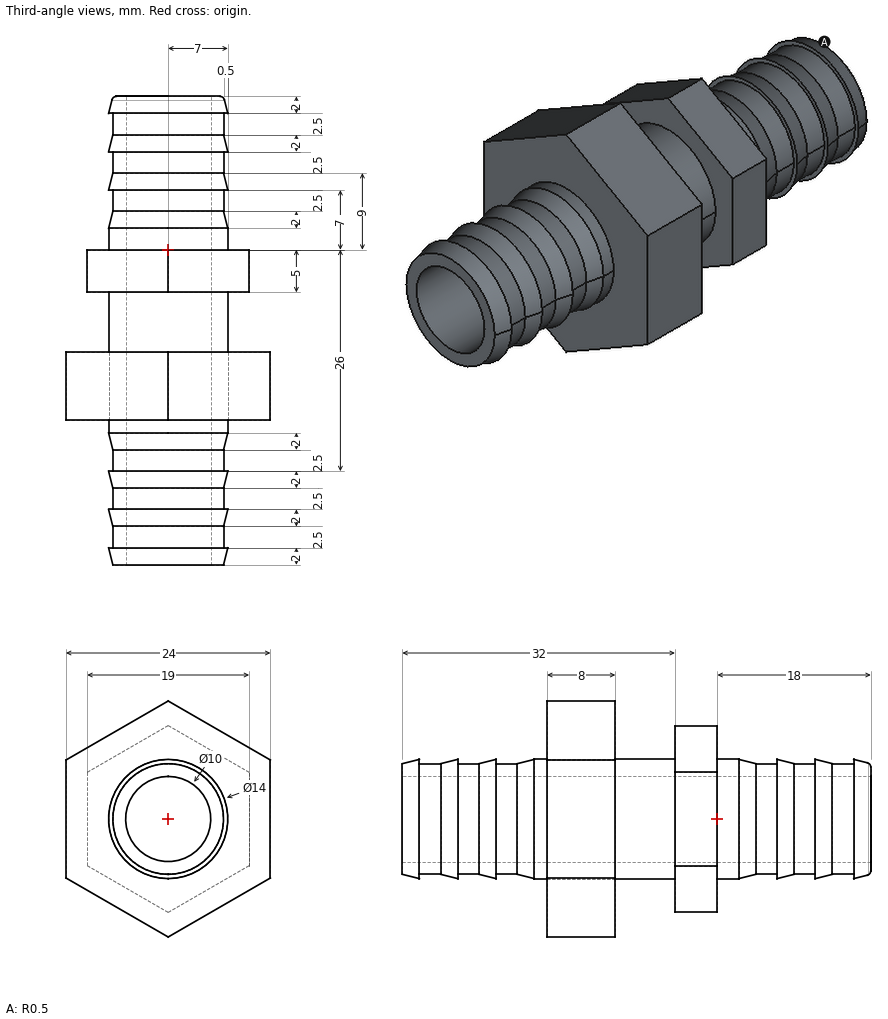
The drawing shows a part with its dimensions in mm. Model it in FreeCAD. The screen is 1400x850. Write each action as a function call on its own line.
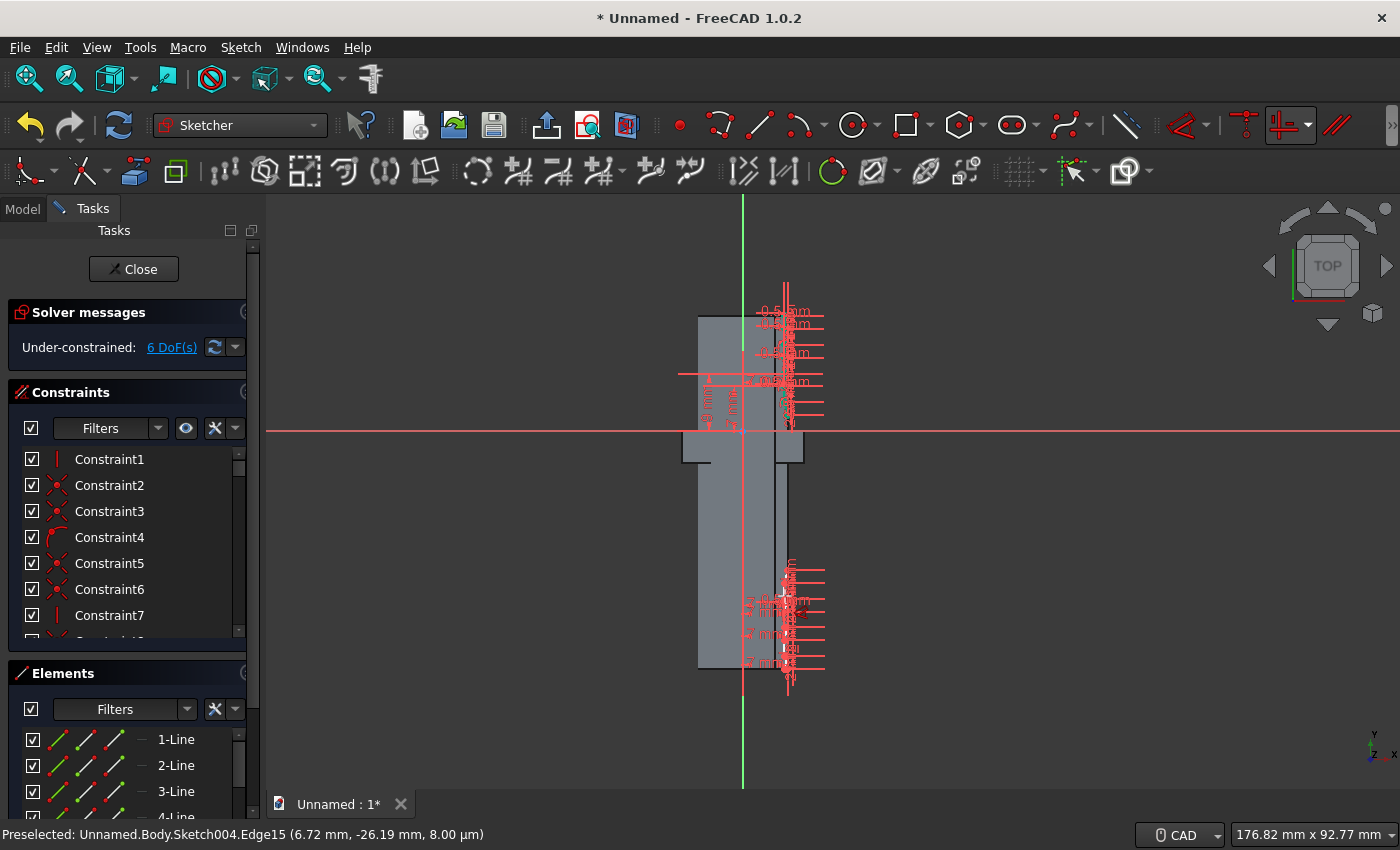
scroll(784, 617, up, 7)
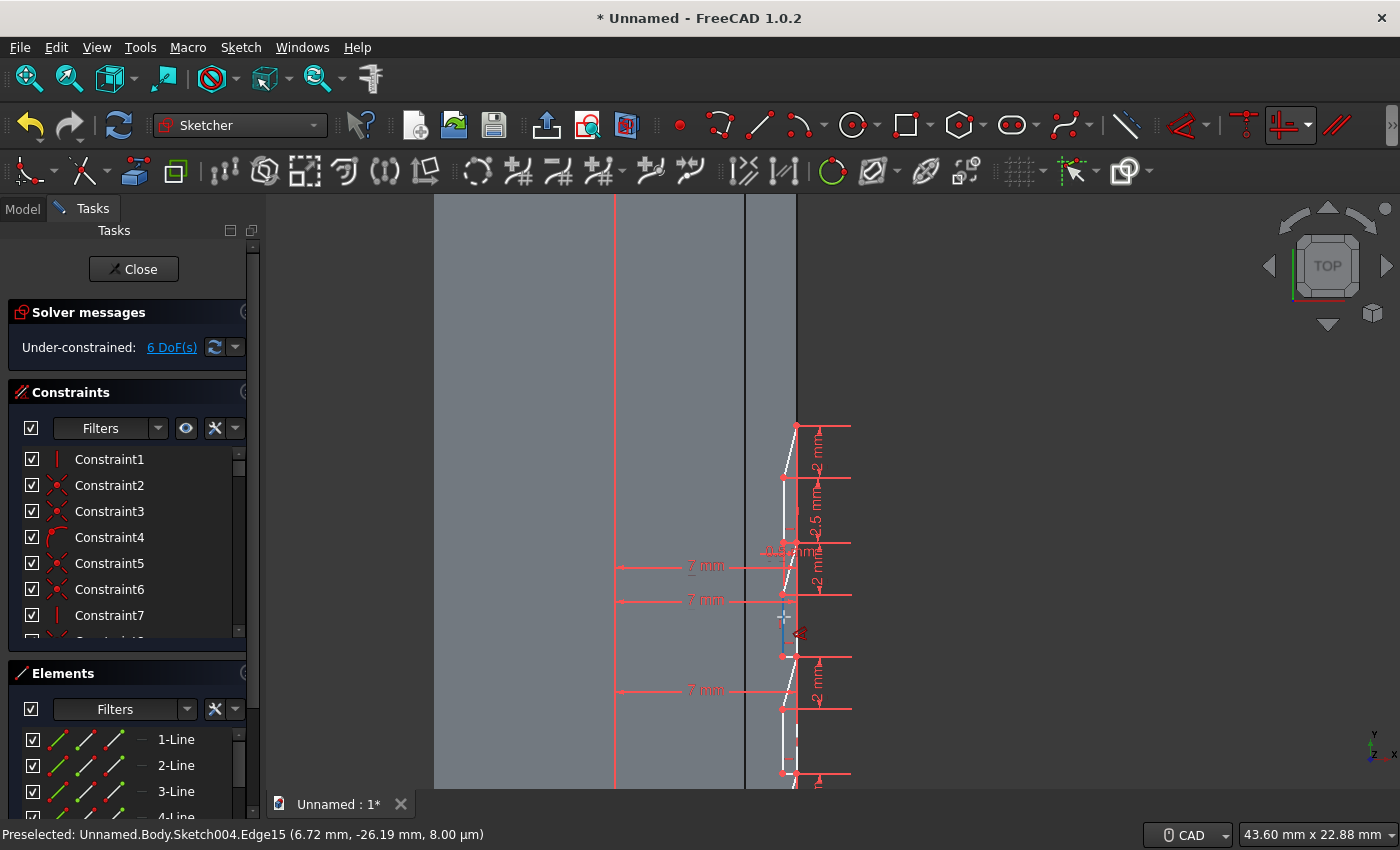
click(783, 614)
click(817, 626)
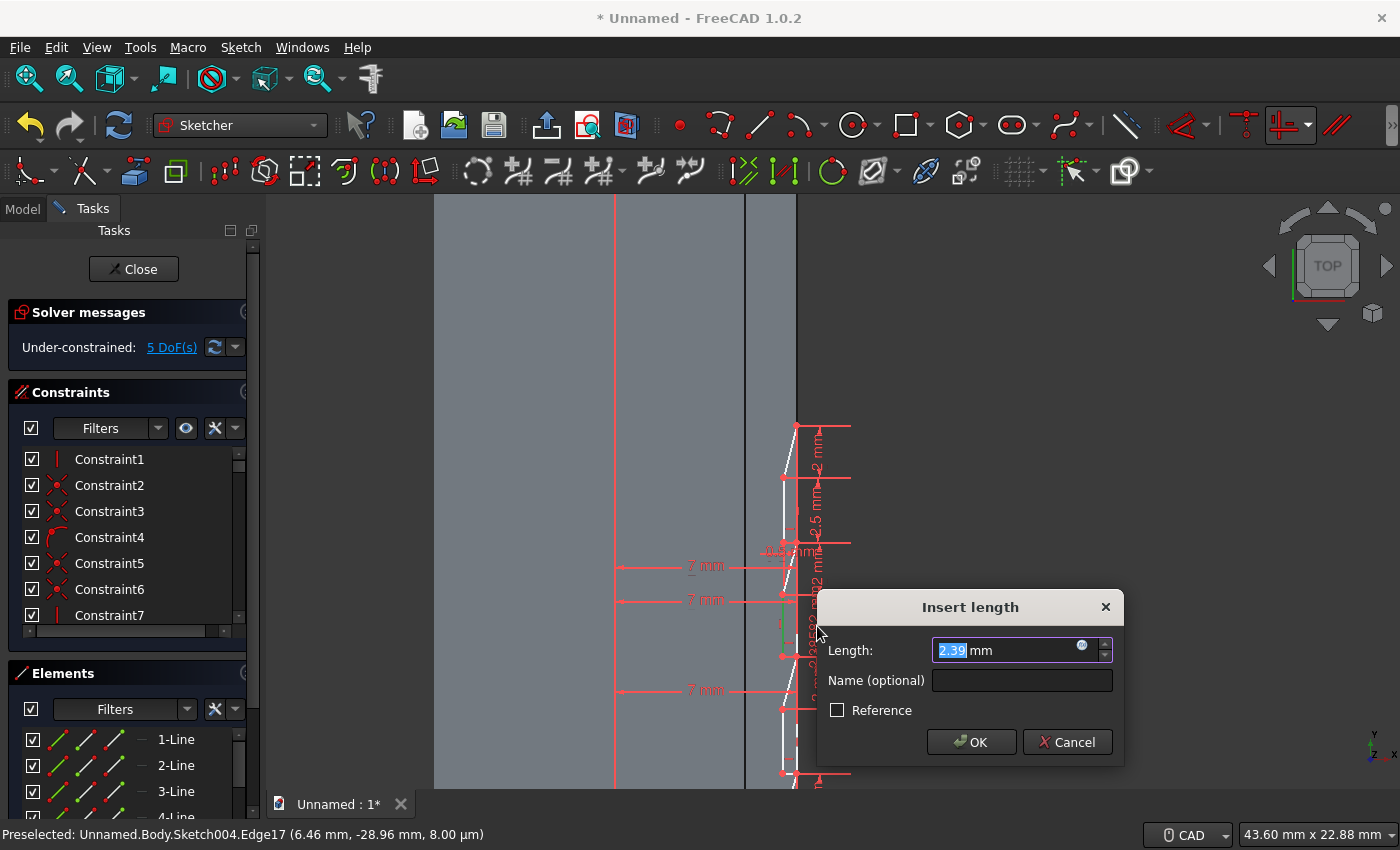
text(2.5)
key(Return)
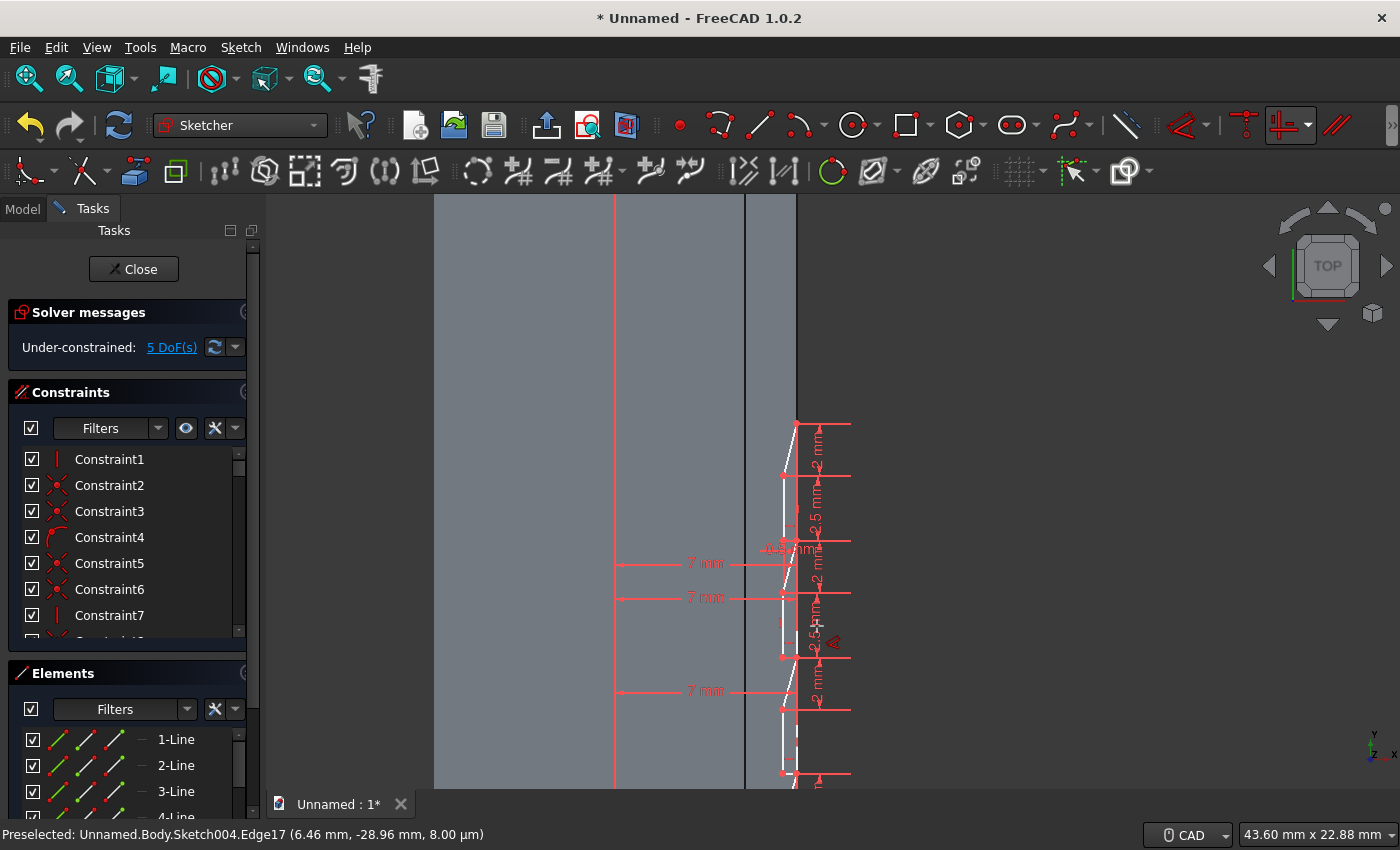
scroll(790, 658, up, 6)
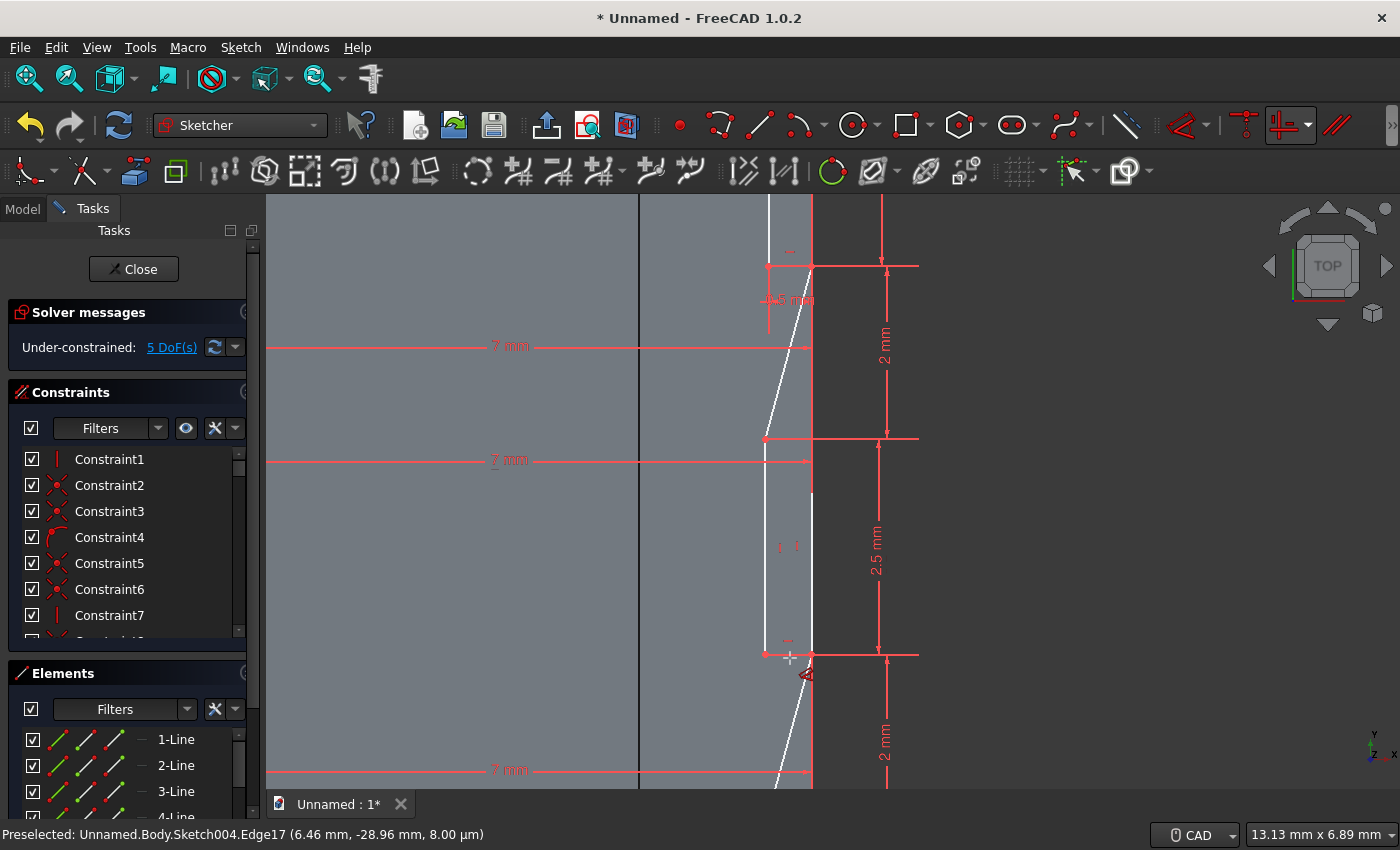
click(789, 655)
click(789, 689)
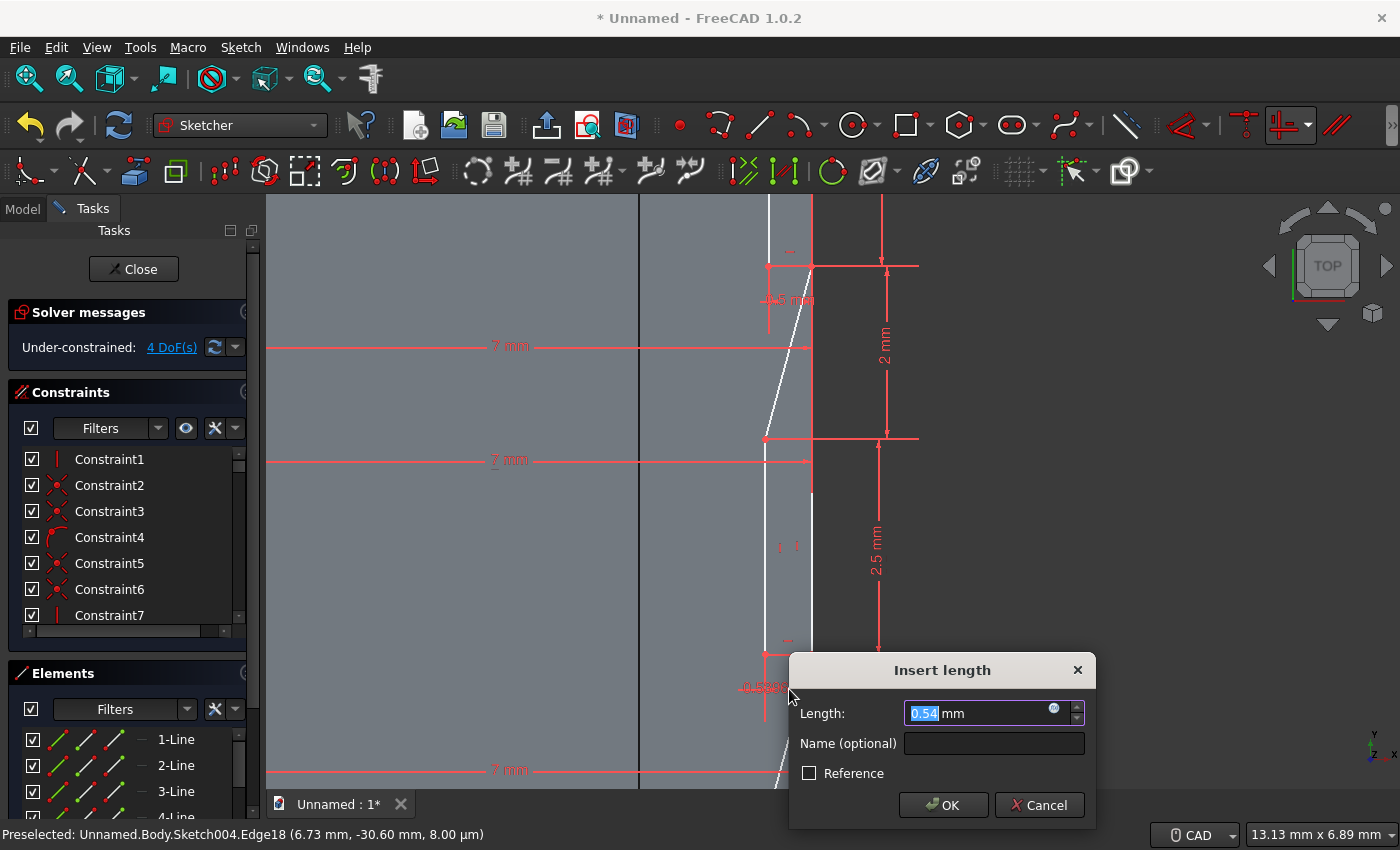
text(0.5)
key(Return)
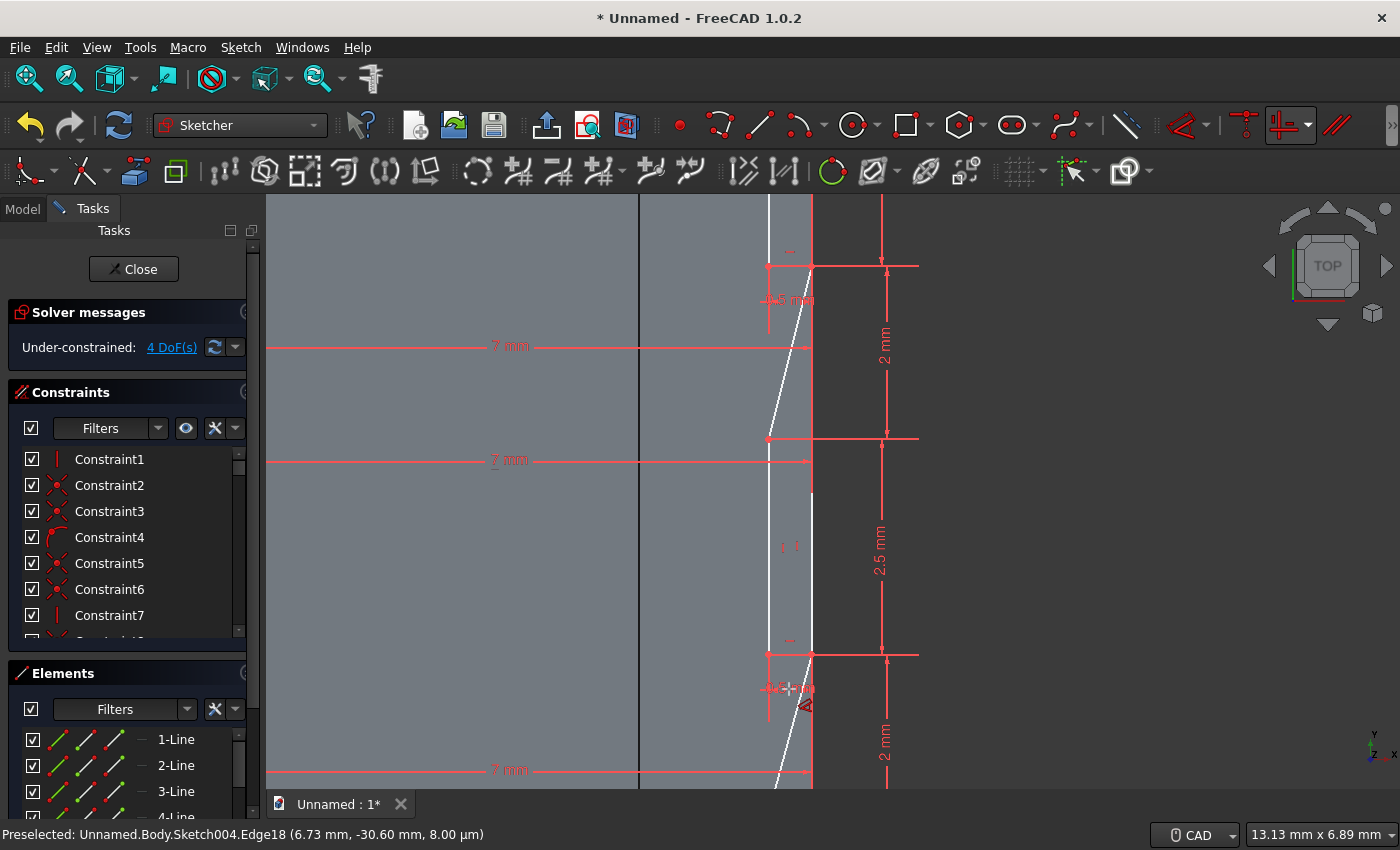
scroll(785, 625, down, 13)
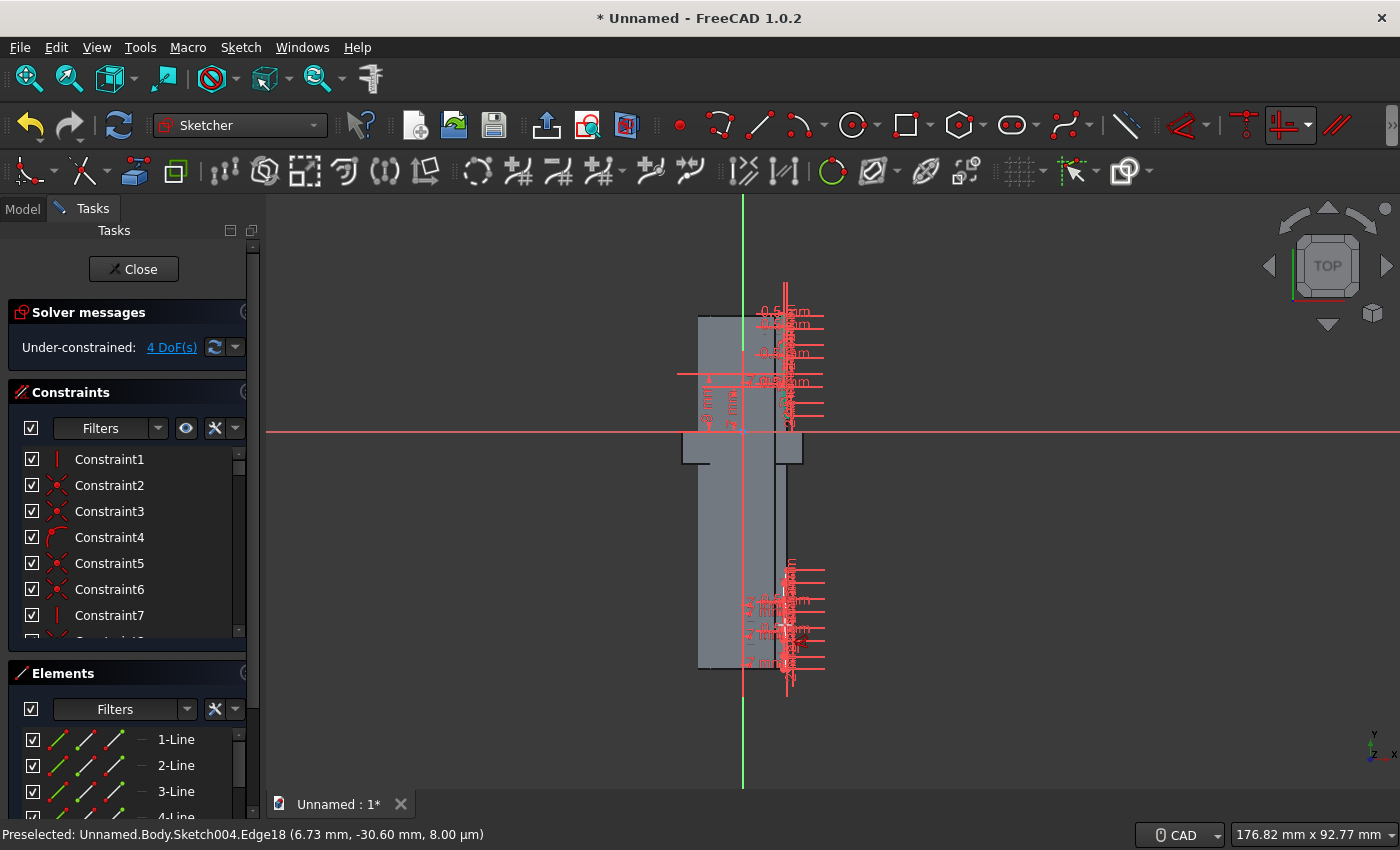
scroll(784, 645, up, 7)